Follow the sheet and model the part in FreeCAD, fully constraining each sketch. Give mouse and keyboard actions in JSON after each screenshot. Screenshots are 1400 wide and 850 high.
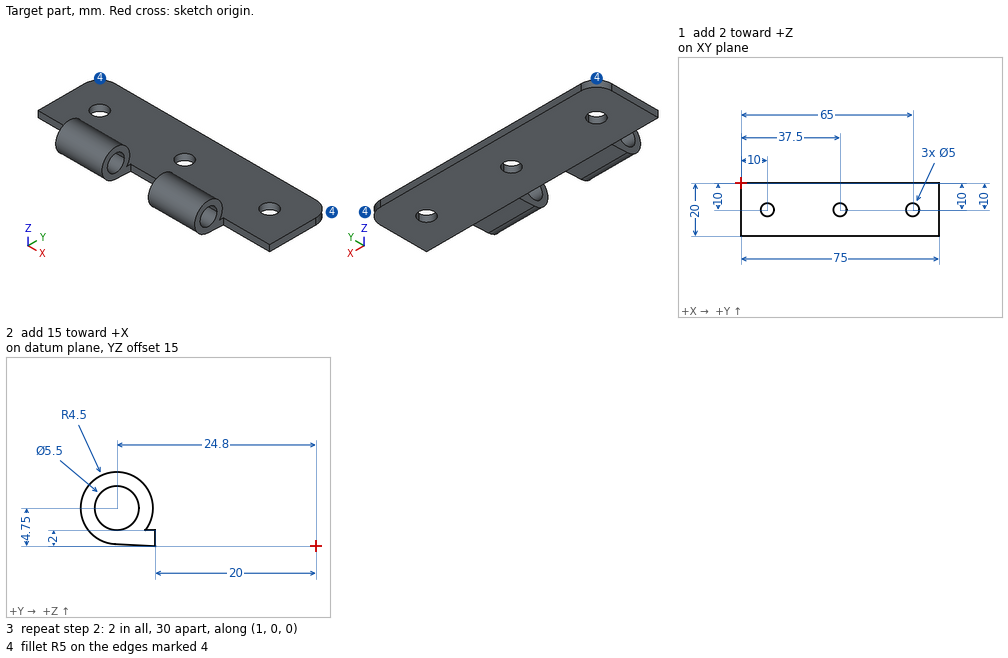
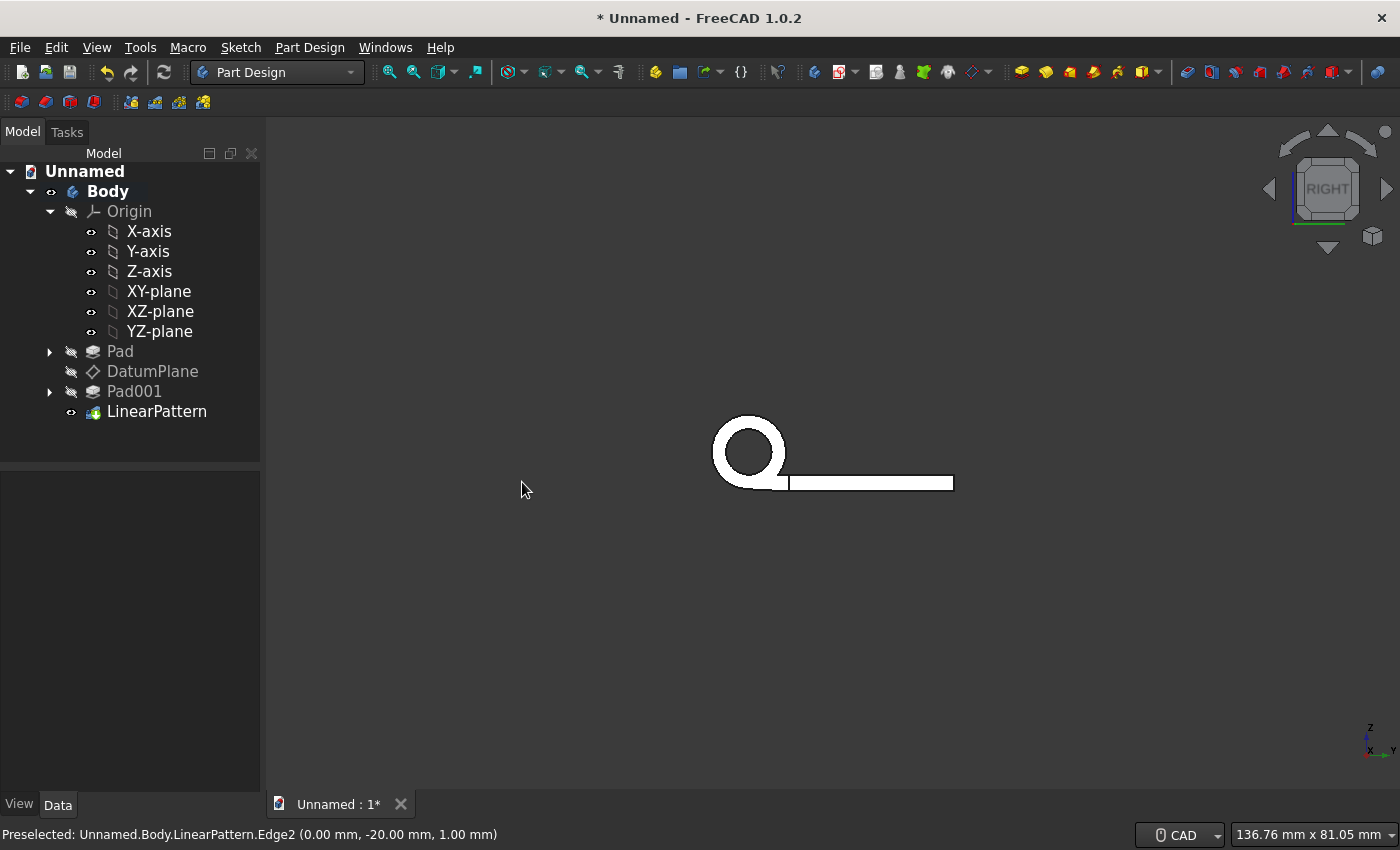
{"action": "left_click", "coordinate": [954, 482]}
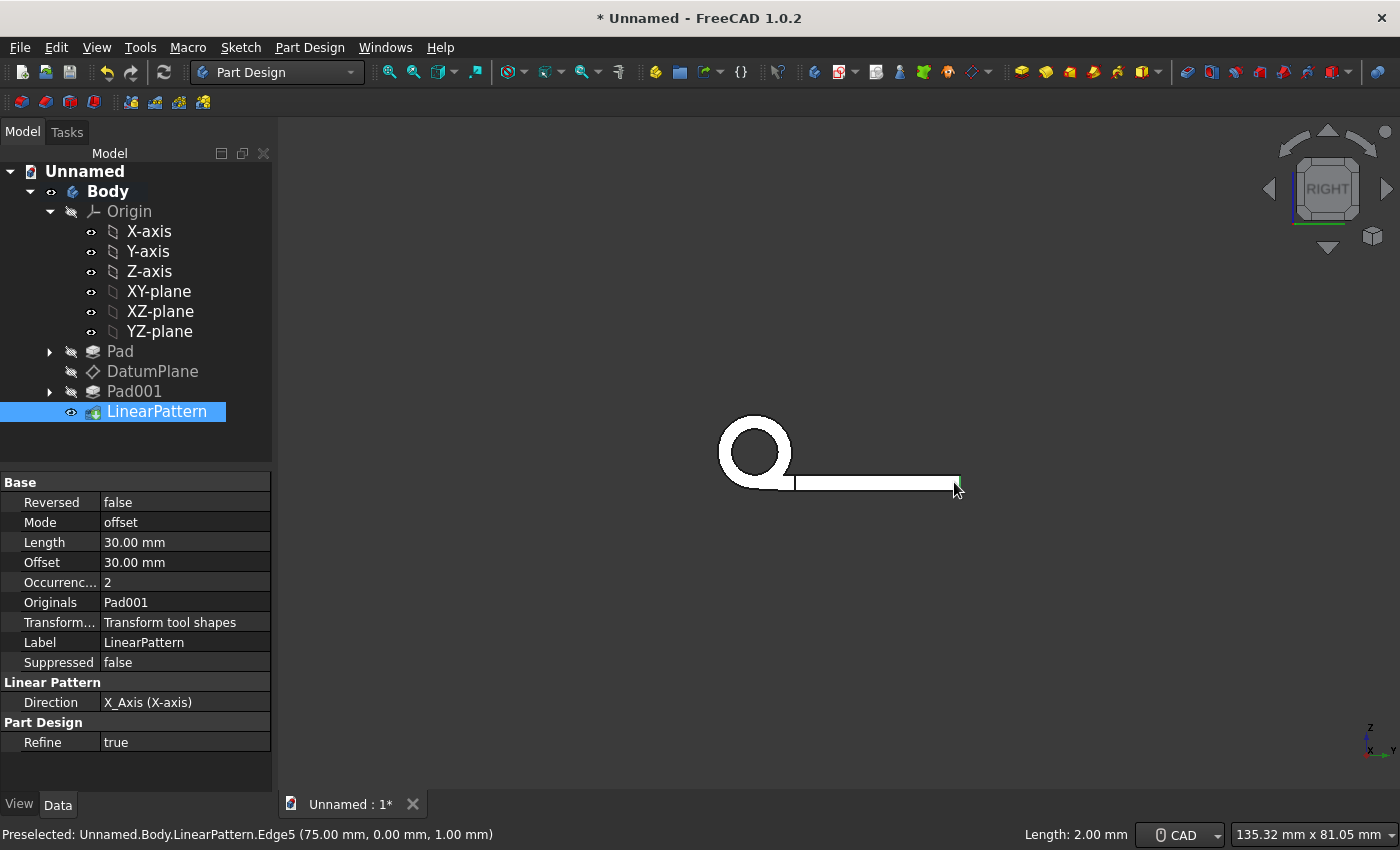
{"action": "scroll", "coordinate": [960, 482], "scroll_direction": "up", "scroll_amount": 5}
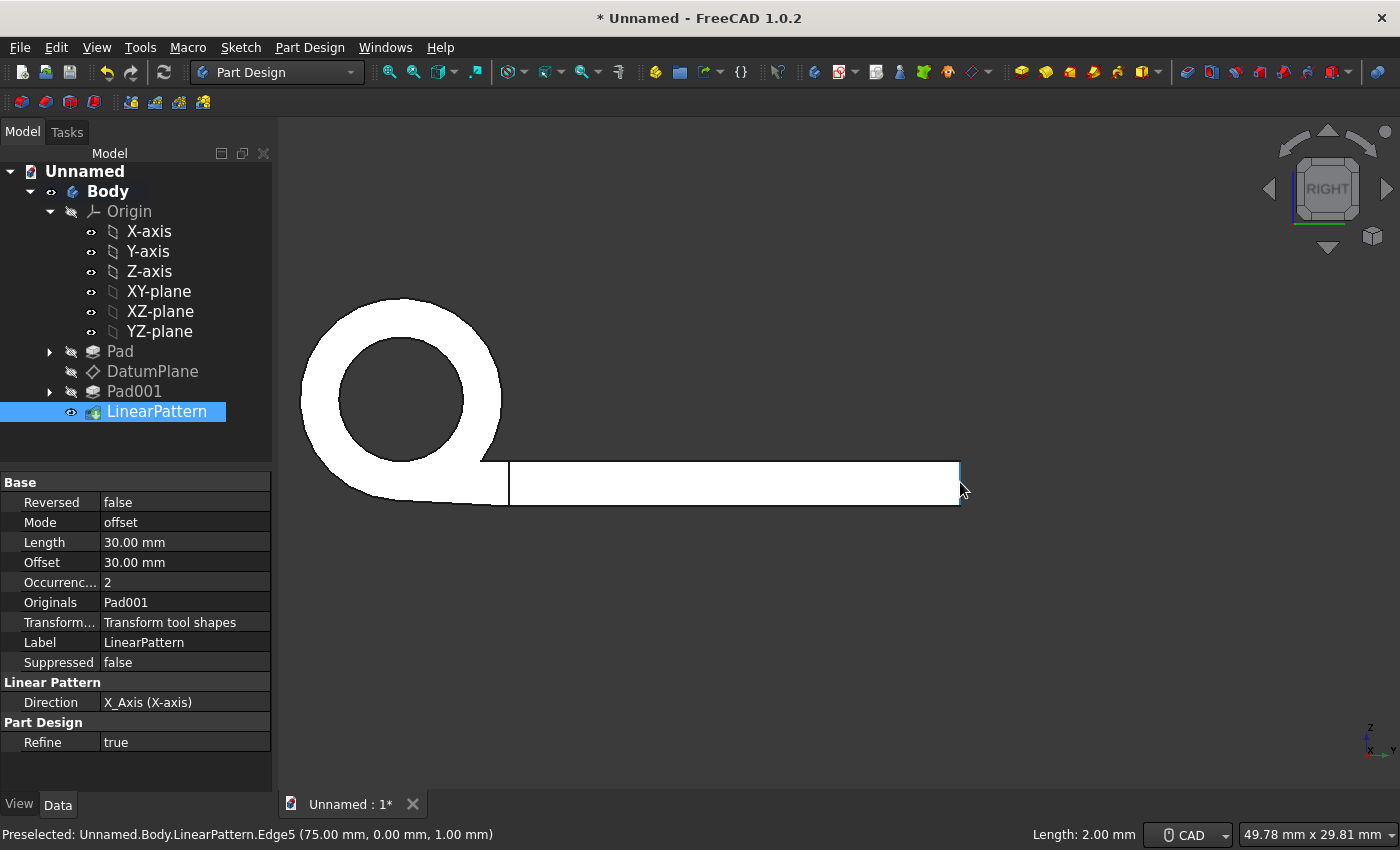
{"action": "key", "text": "v f"}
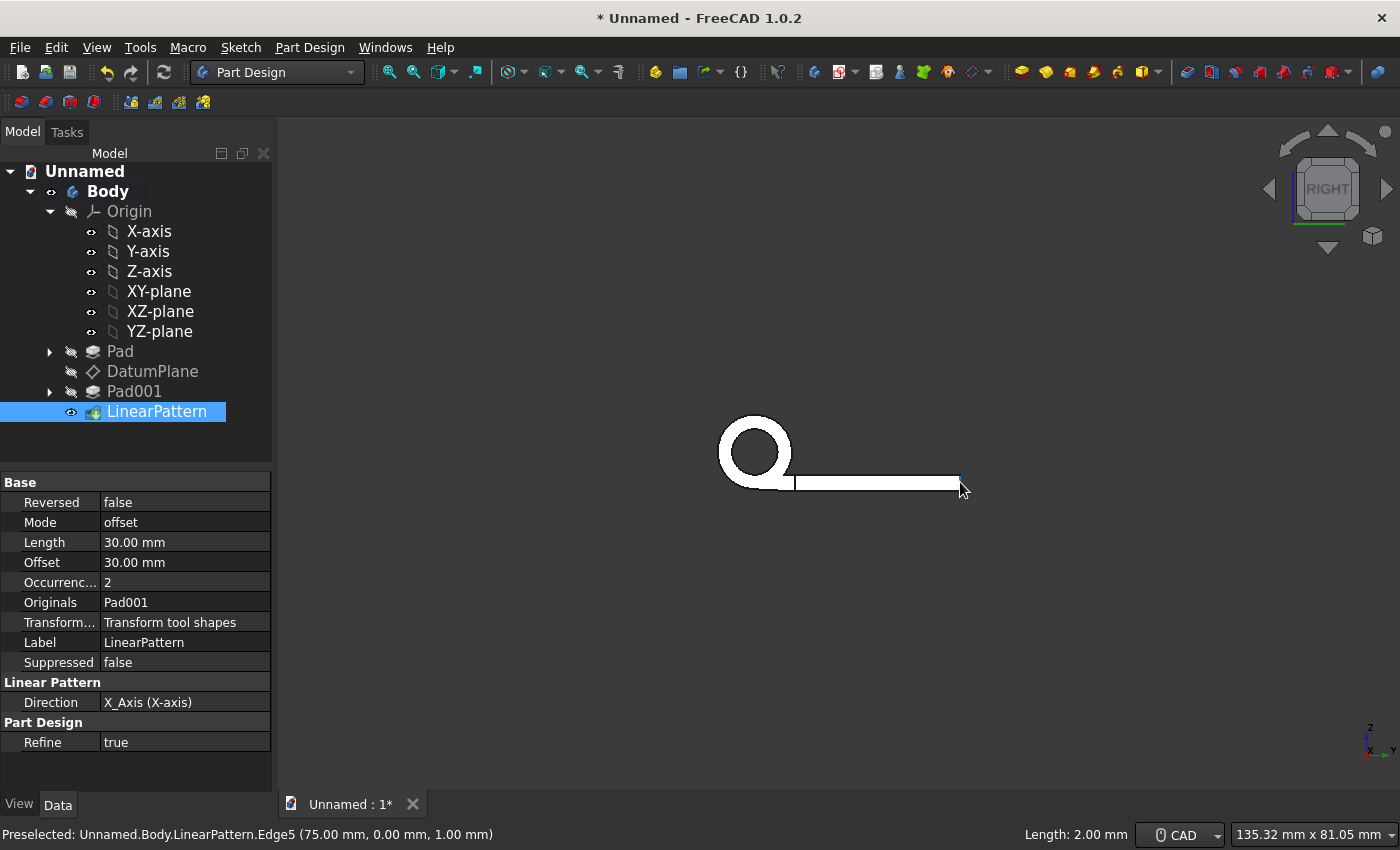
{"action": "key", "text": "5"}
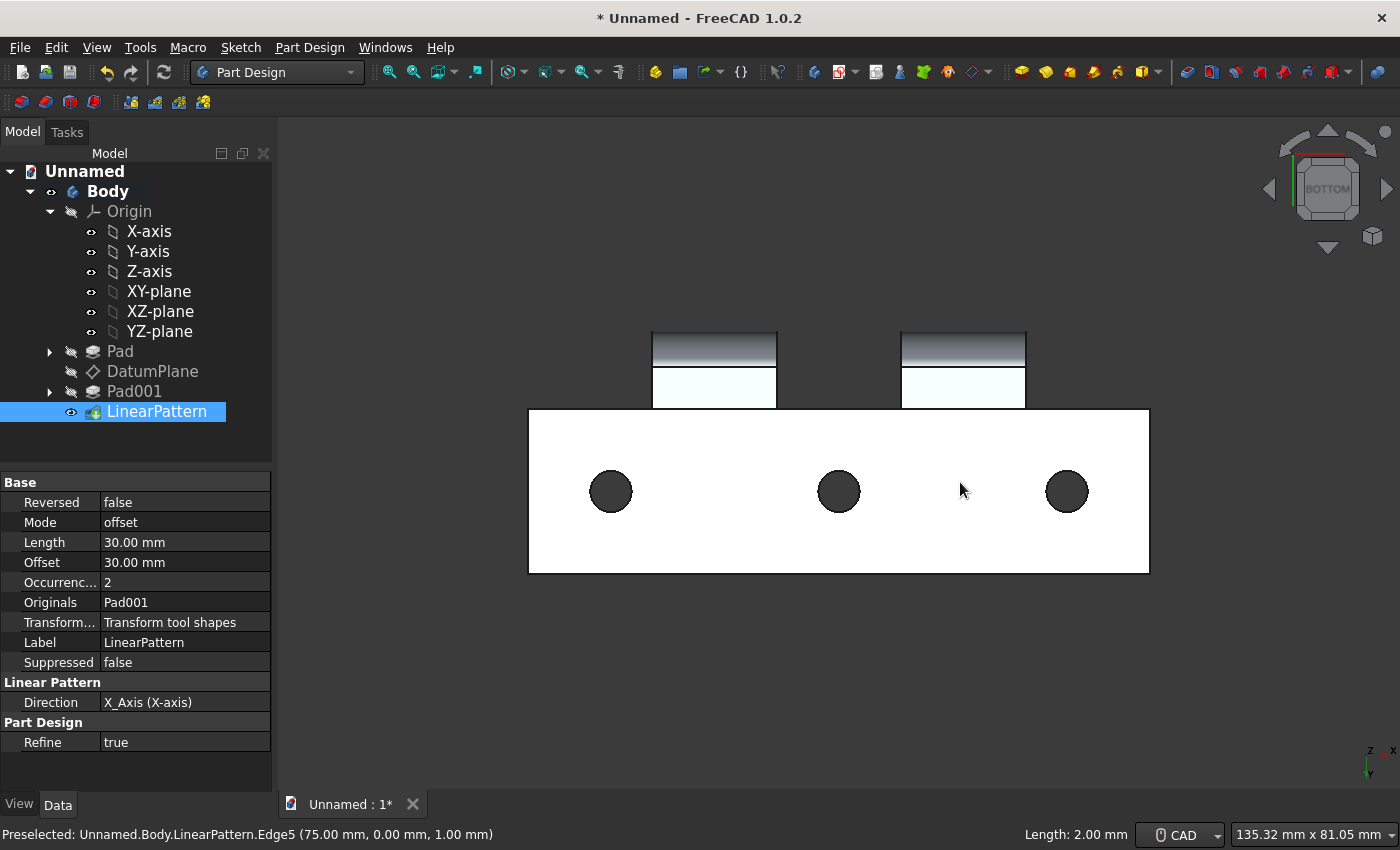
{"action": "scroll", "coordinate": [528, 573], "scroll_direction": "up", "scroll_amount": 5}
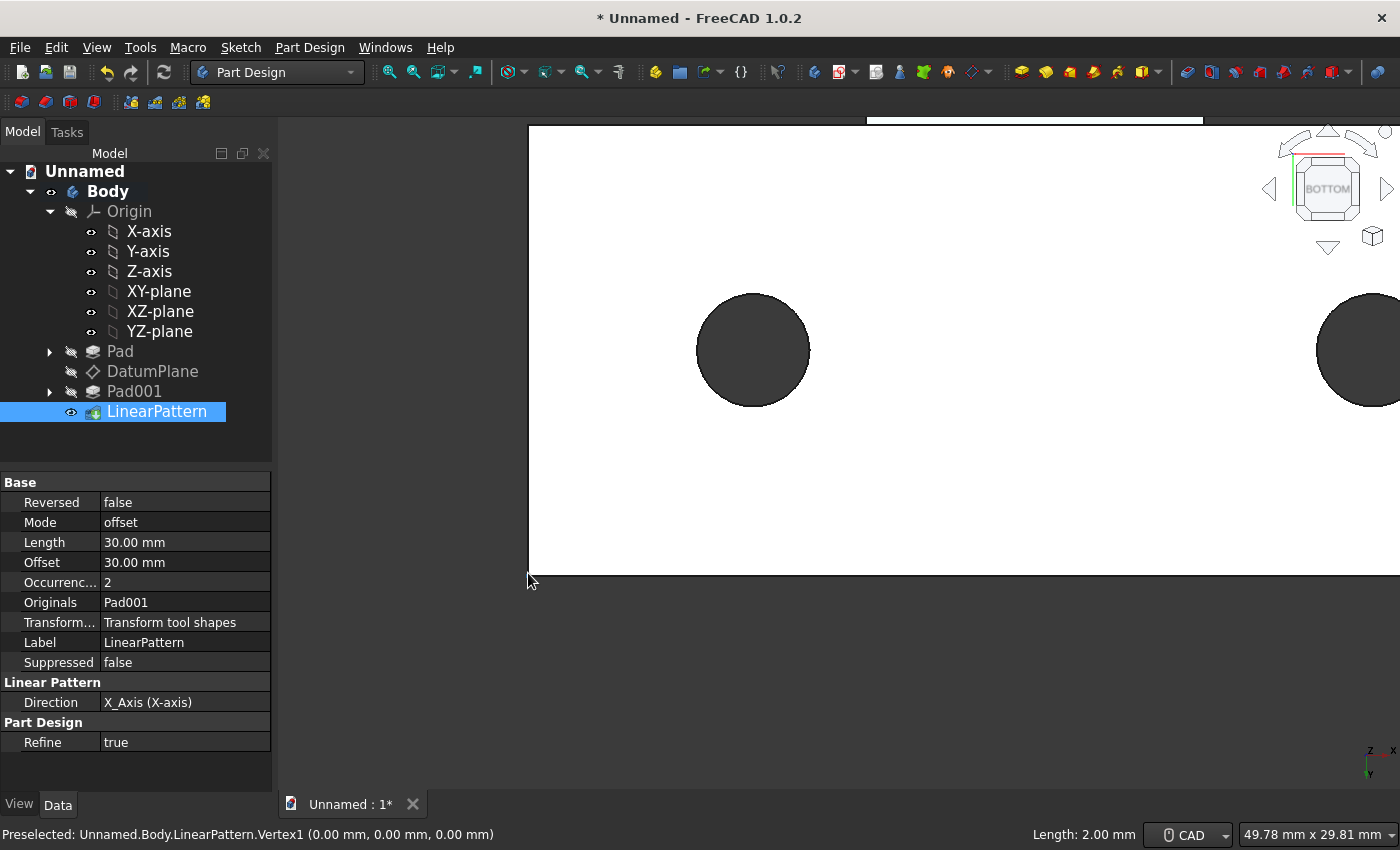
{"action": "key", "text": "v f"}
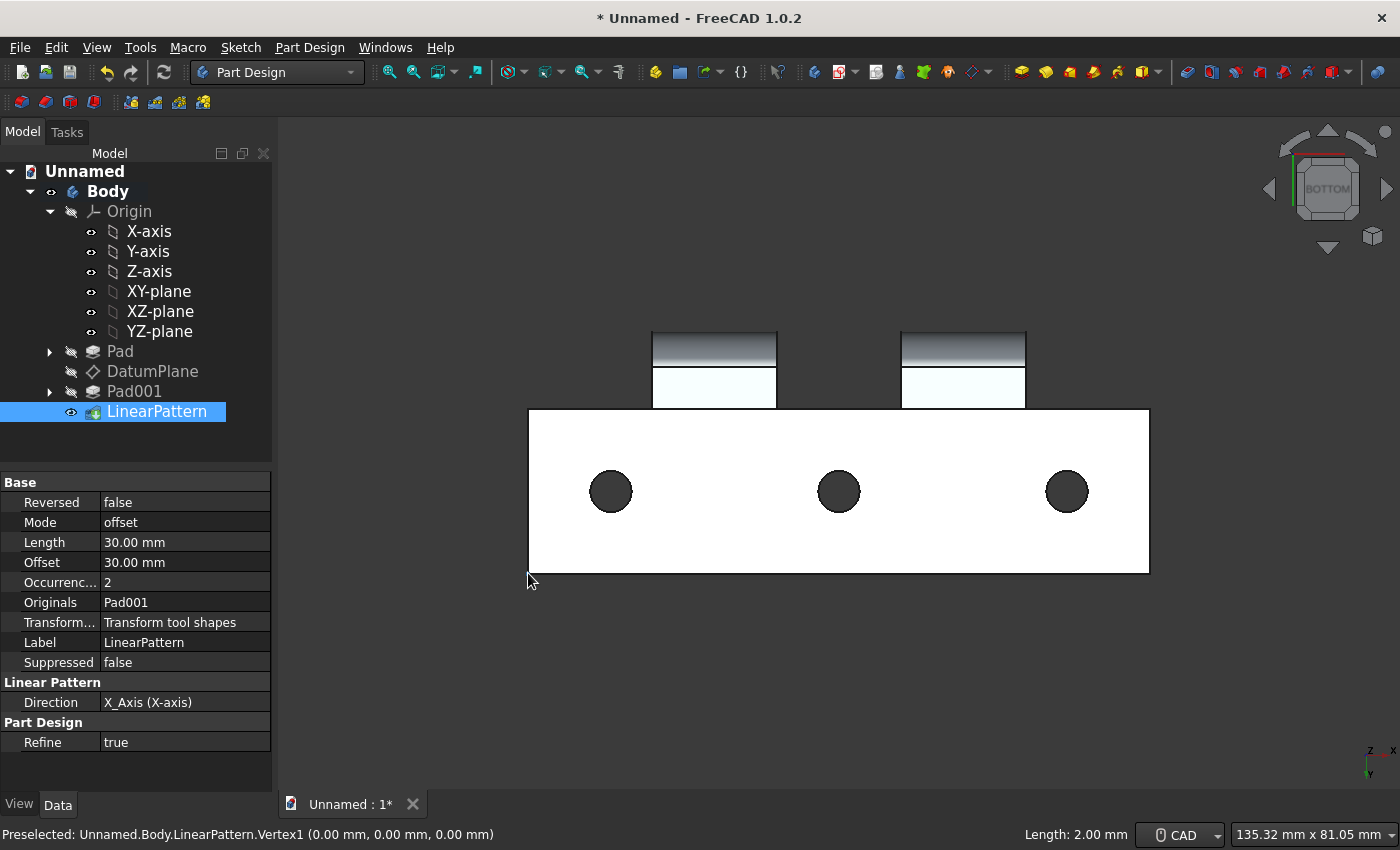
{"action": "key", "text": "4"}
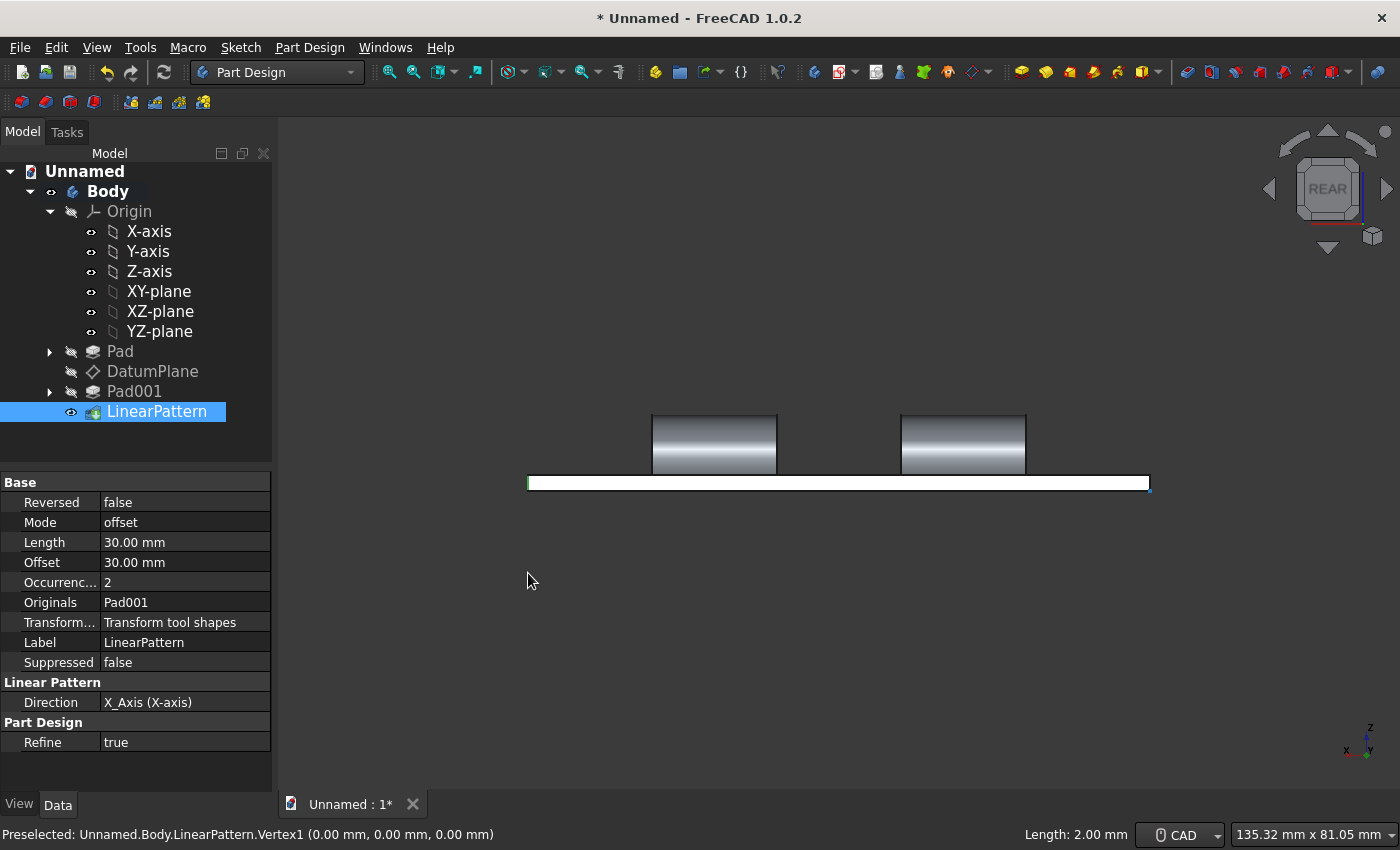
{"action": "left_click", "coordinate": [1150, 482], "text": "ctrl"}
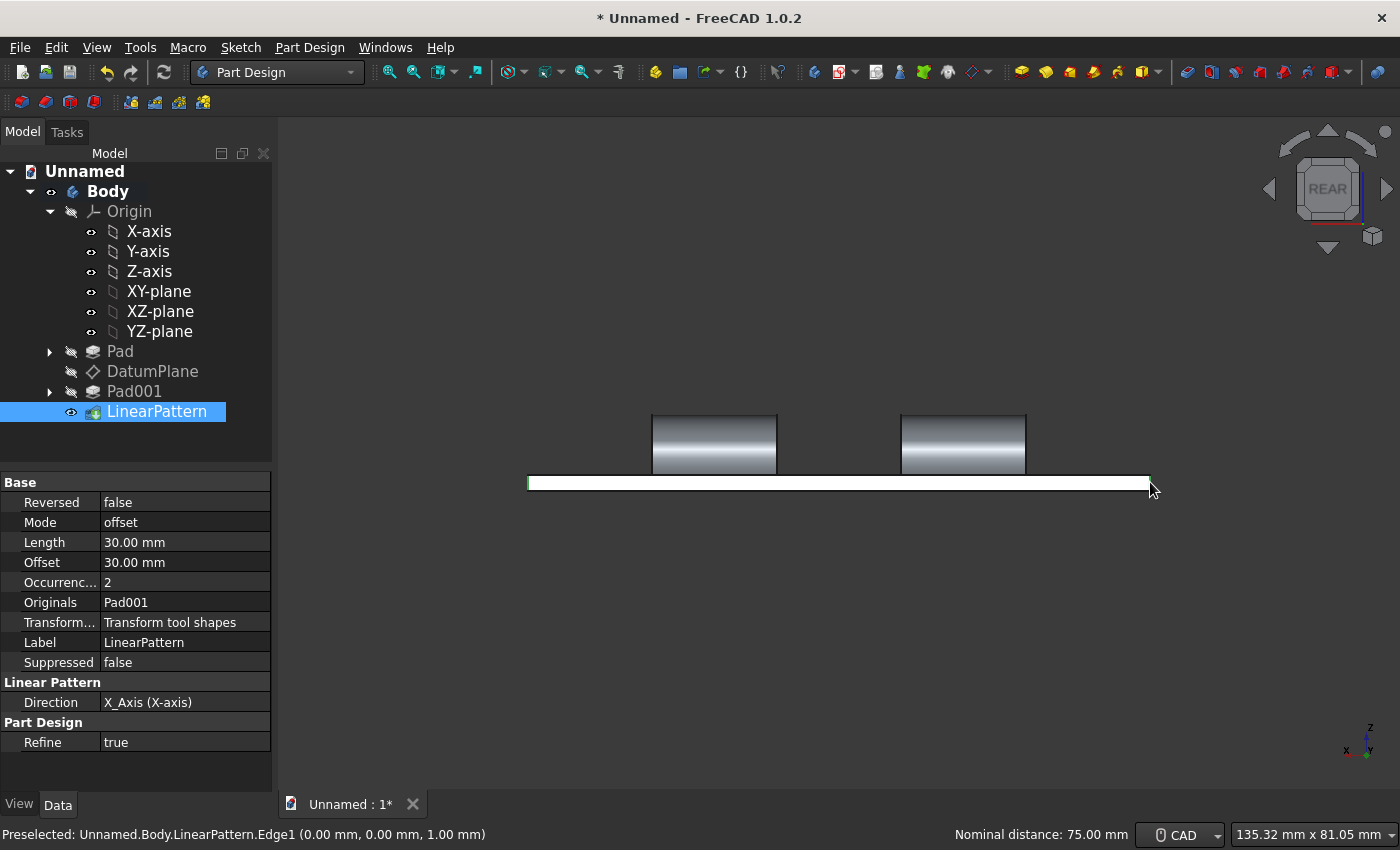
{"action": "left_click", "coordinate": [22, 102]}